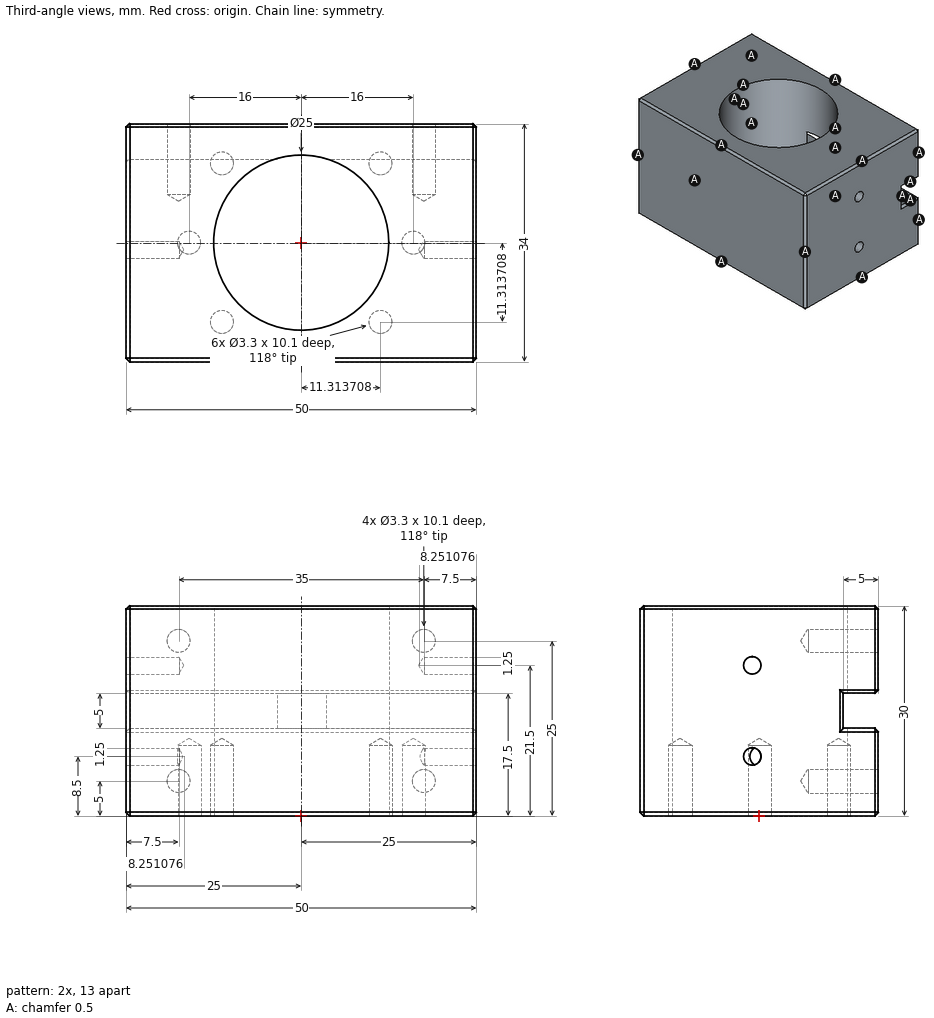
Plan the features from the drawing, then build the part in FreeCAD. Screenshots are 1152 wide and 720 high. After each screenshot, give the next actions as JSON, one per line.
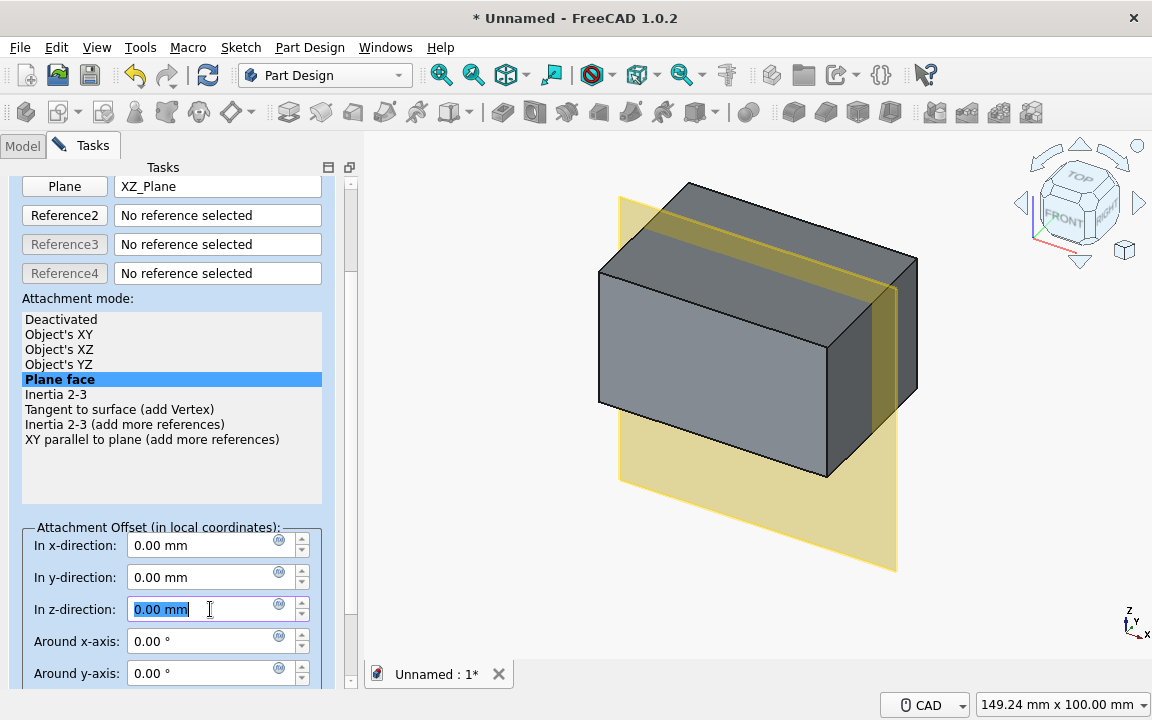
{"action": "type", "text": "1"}
{"action": "key", "text": "Tab"}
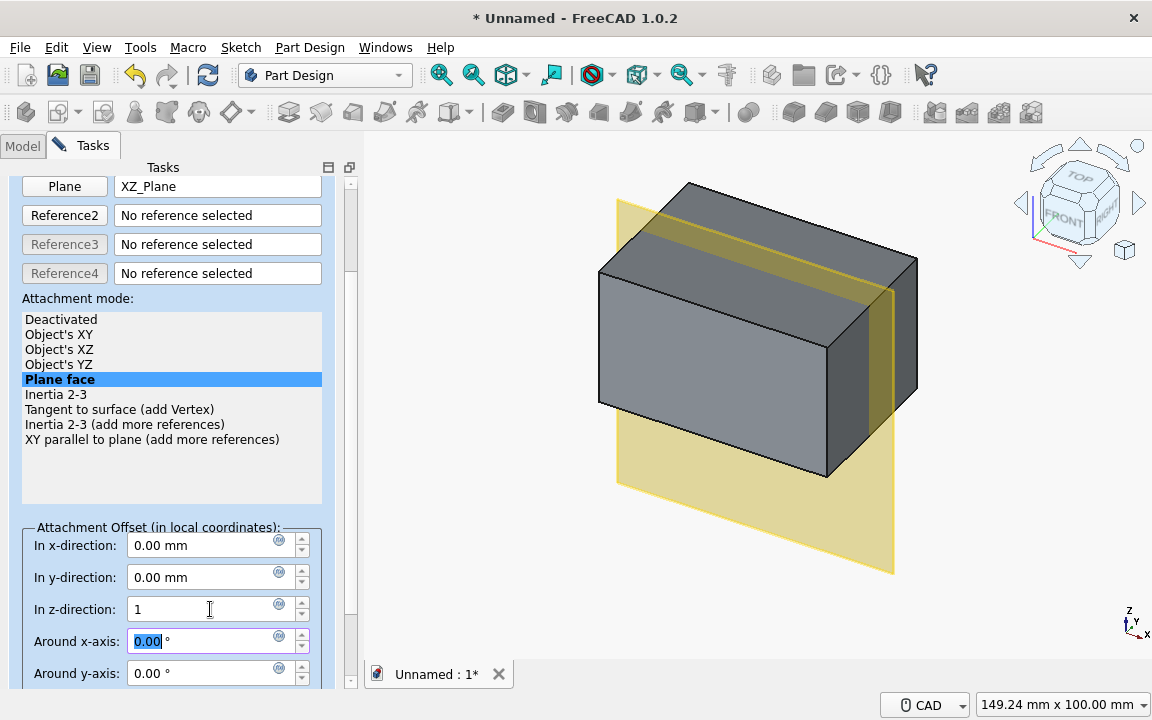
{"action": "scroll", "coordinate": [351, 432], "scroll_direction": "up", "scroll_amount": 3}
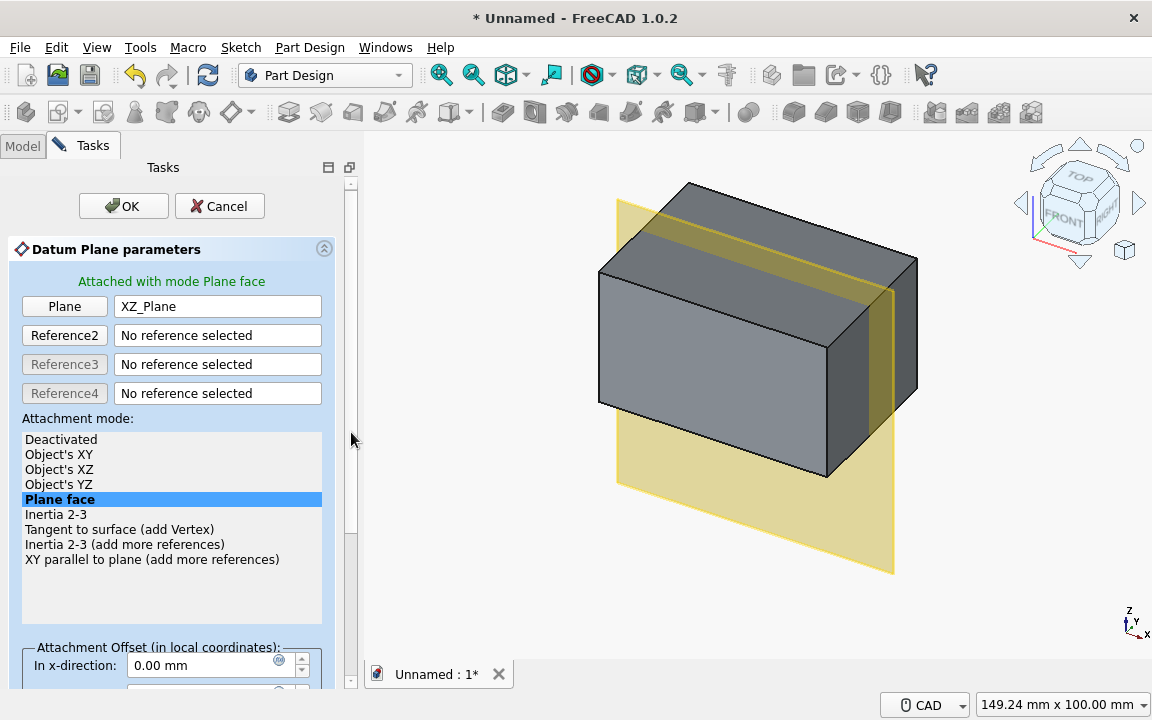
{"action": "left_click", "coordinate": [124, 206]}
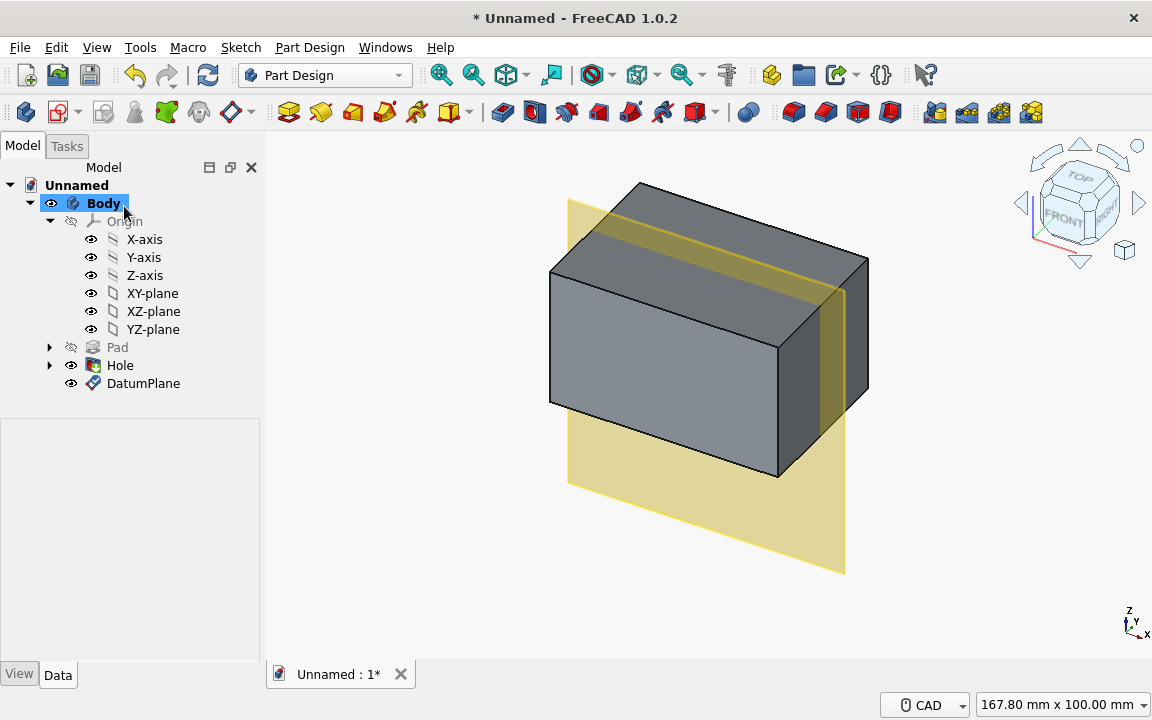
{"action": "left_click", "coordinate": [116, 383]}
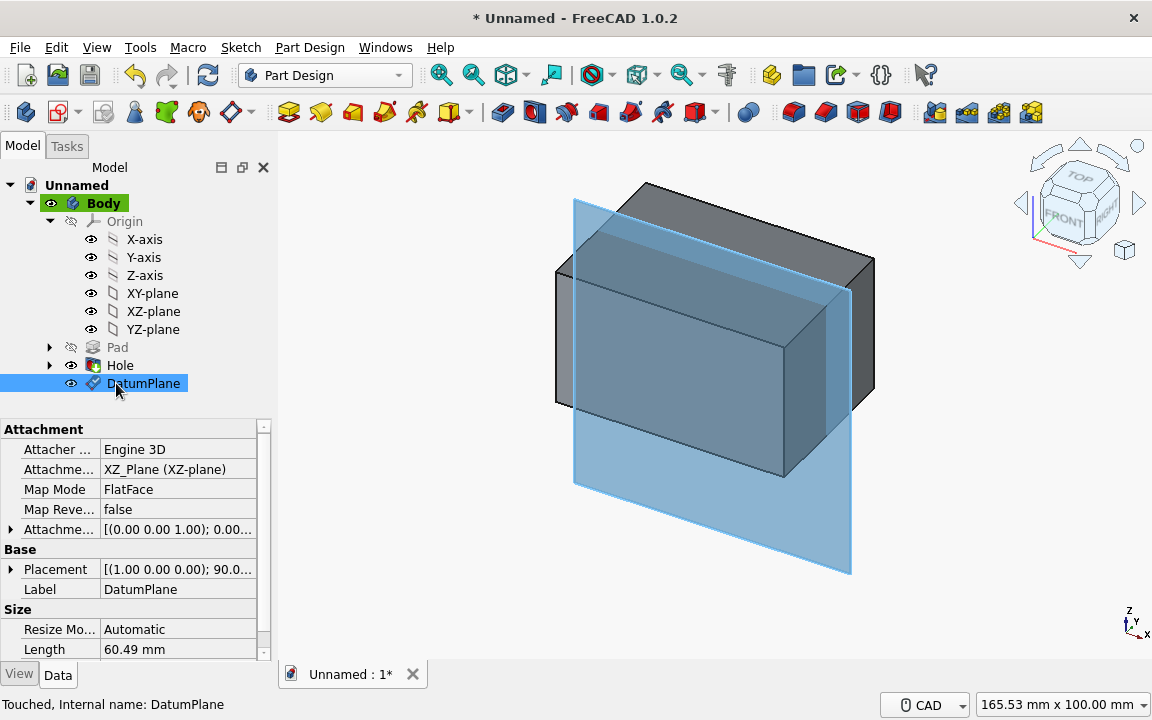
{"action": "left_click", "coordinate": [58, 112]}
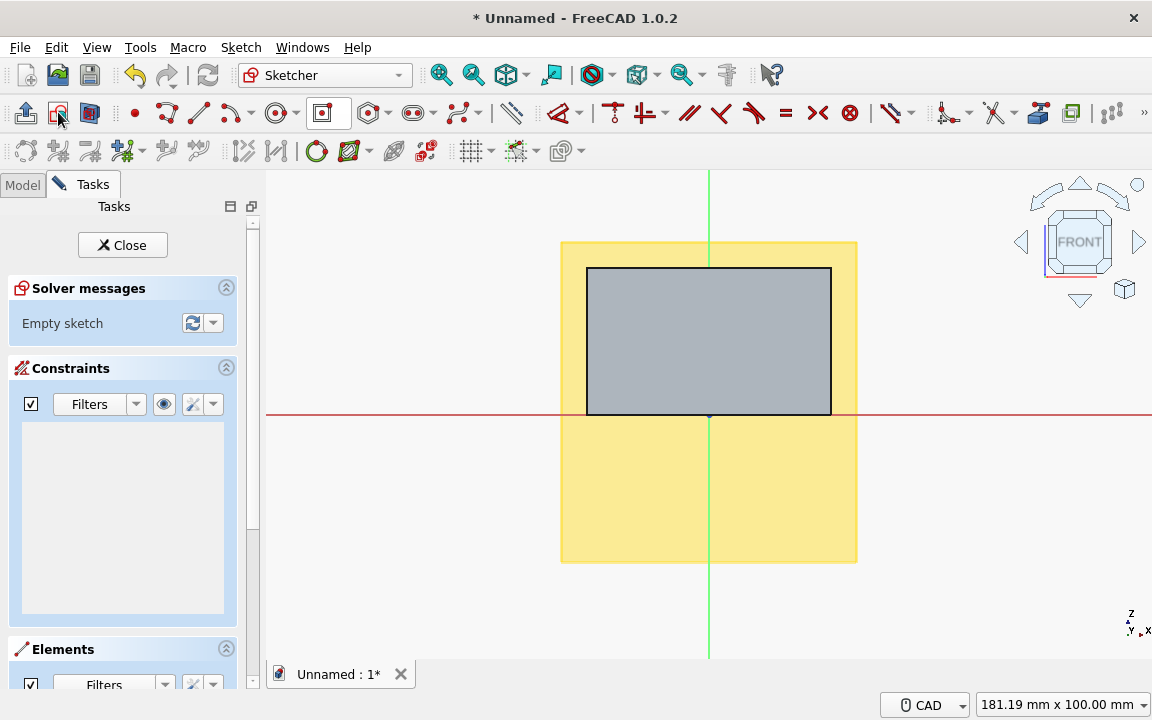
{"action": "key", "text": "q s"}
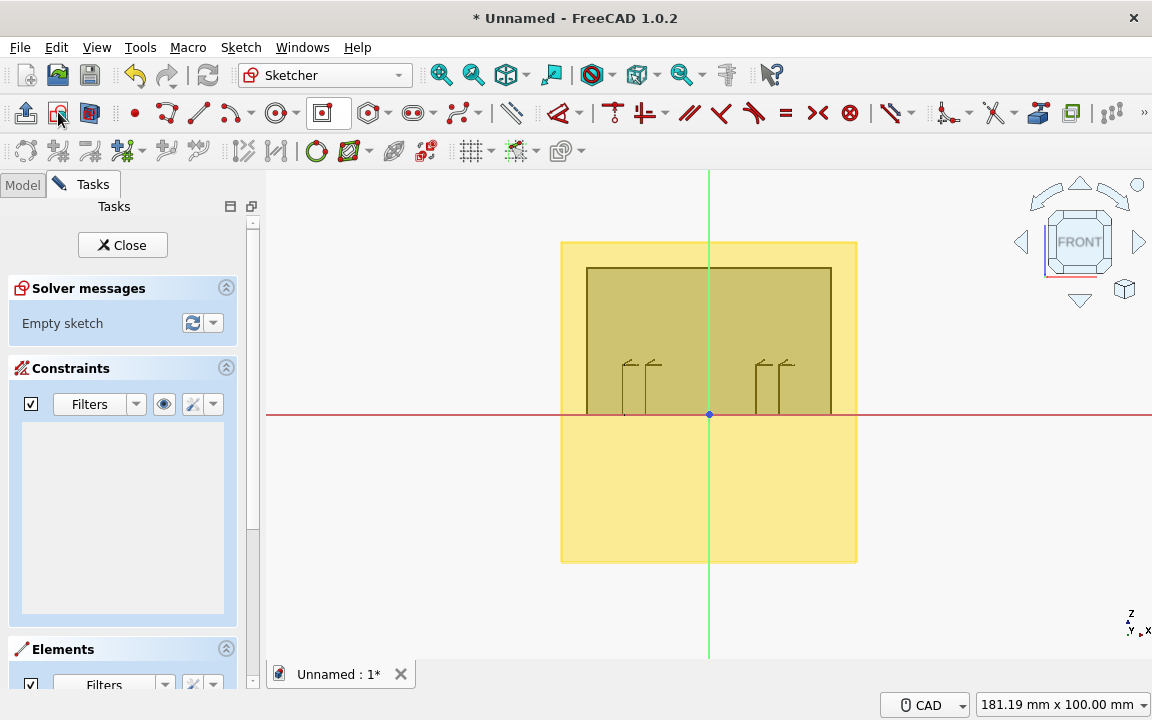
{"action": "scroll", "coordinate": [650, 383], "scroll_direction": "up", "scroll_amount": 7}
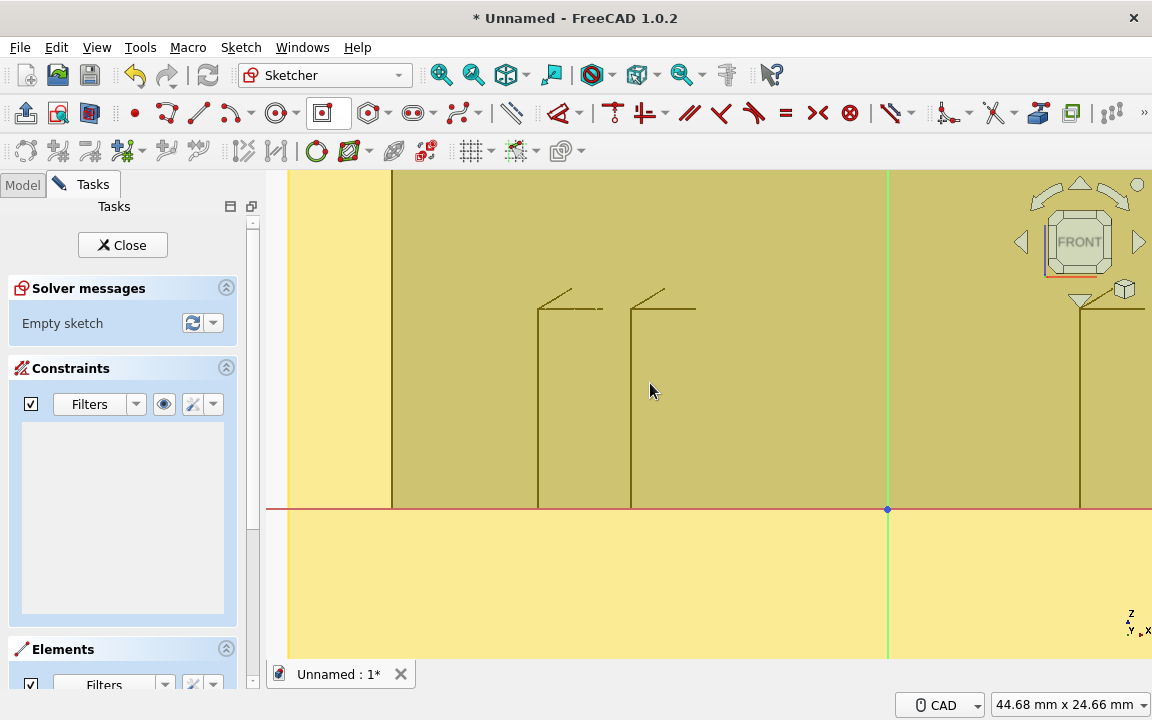
{"action": "key", "text": "g m"}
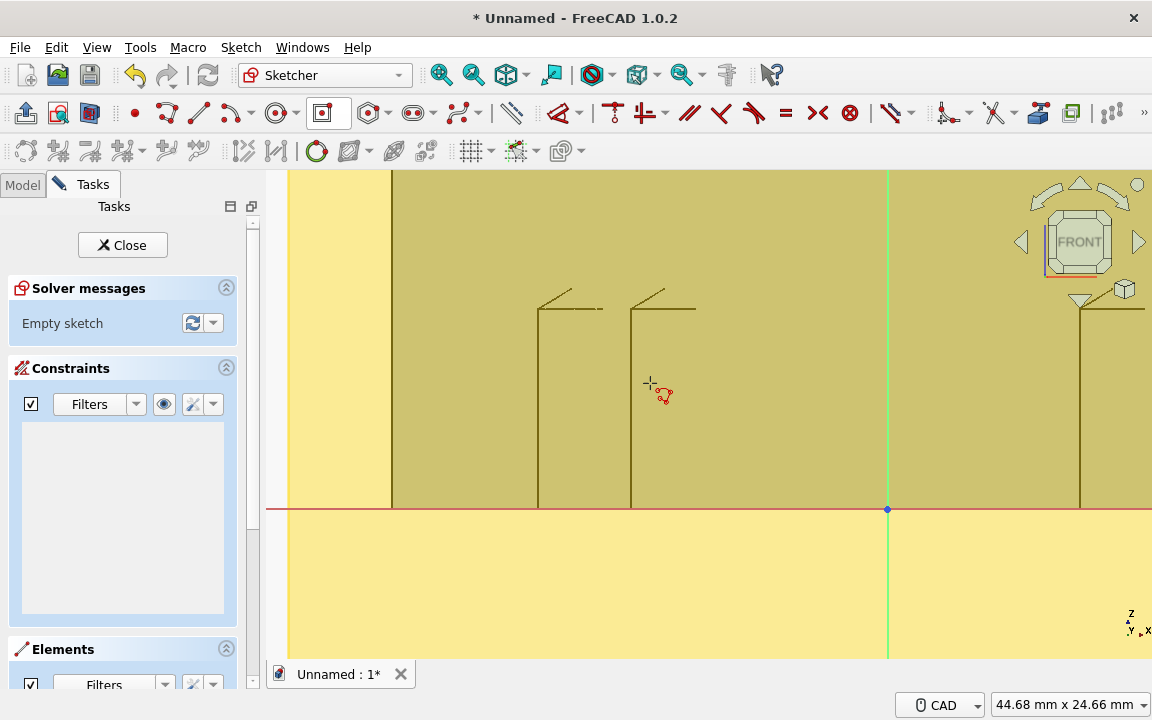
{"action": "left_click", "coordinate": [556, 341]}
{"action": "left_click", "coordinate": [392, 341]}
{"action": "left_click", "coordinate": [392, 316]}
{"action": "left_click", "coordinate": [541, 316]}
{"action": "left_click", "coordinate": [556, 342]}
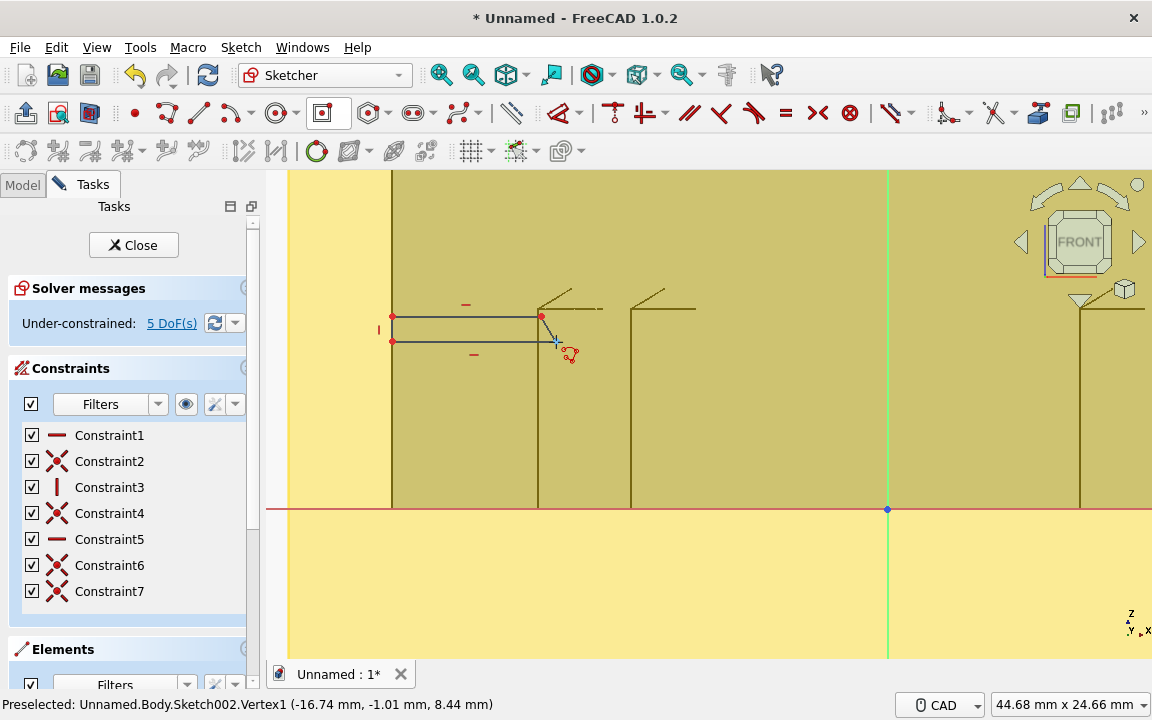
{"action": "left_click", "coordinate": [200, 114]}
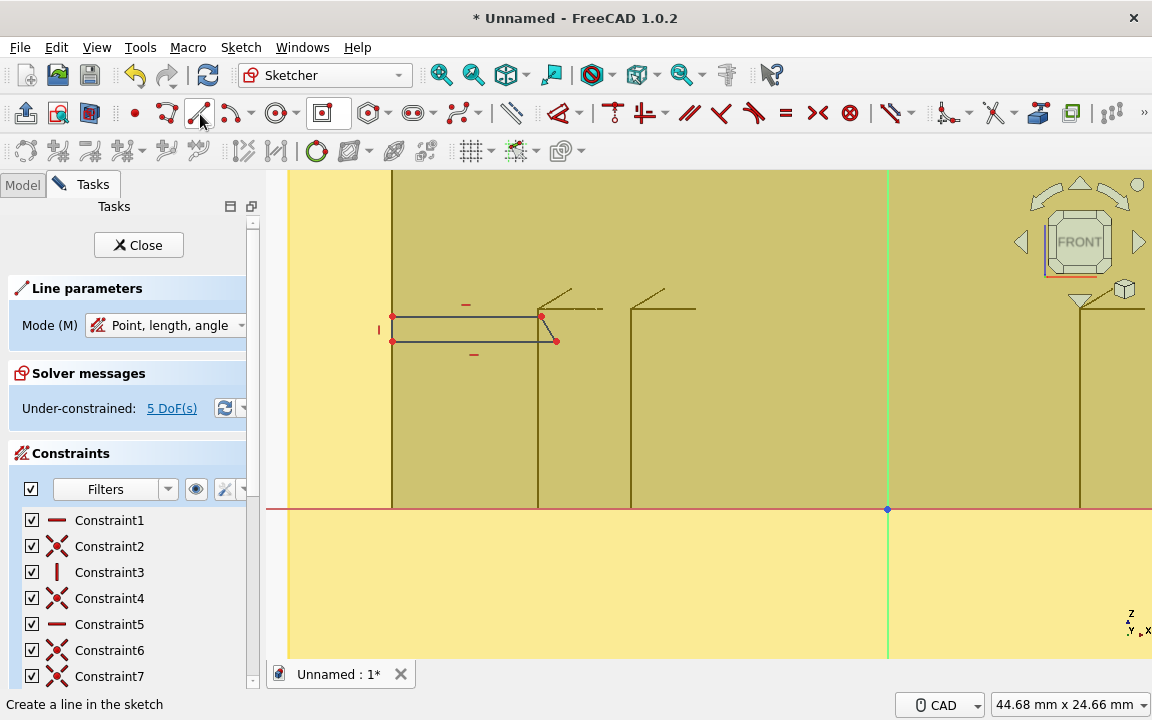
{"action": "left_click", "coordinate": [572, 341]}
{"action": "left_click", "coordinate": [621, 341]}
{"action": "key", "text": "Escape"}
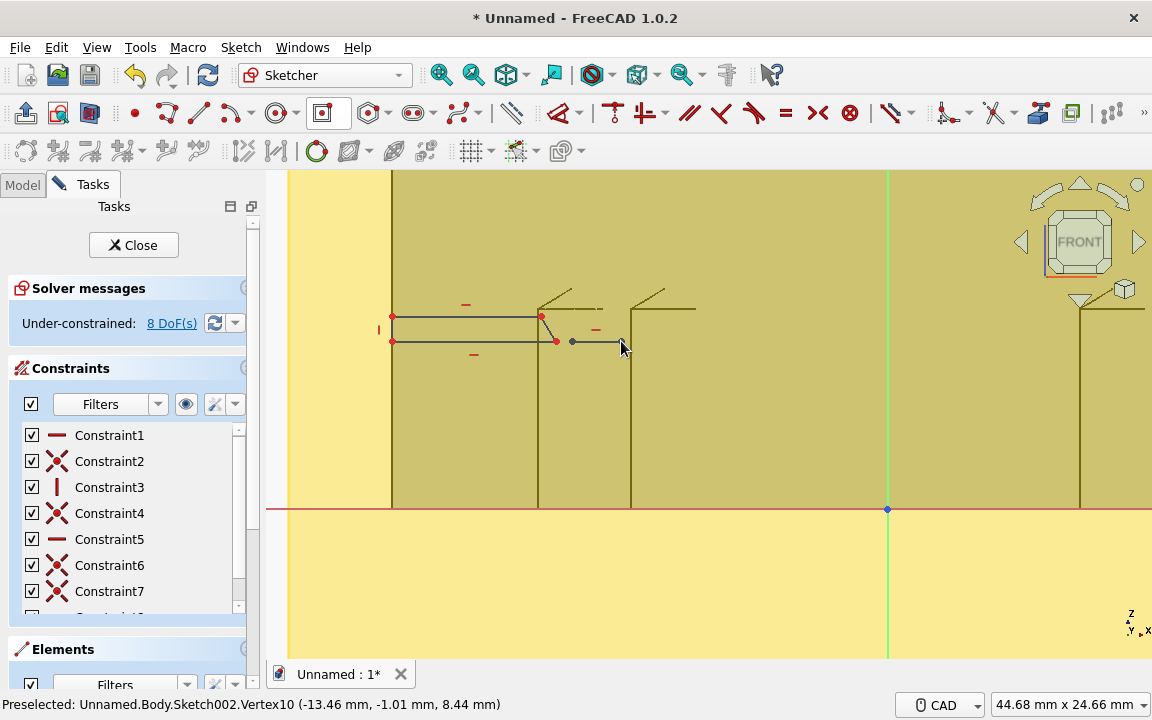
{"action": "left_click", "coordinate": [587, 342]}